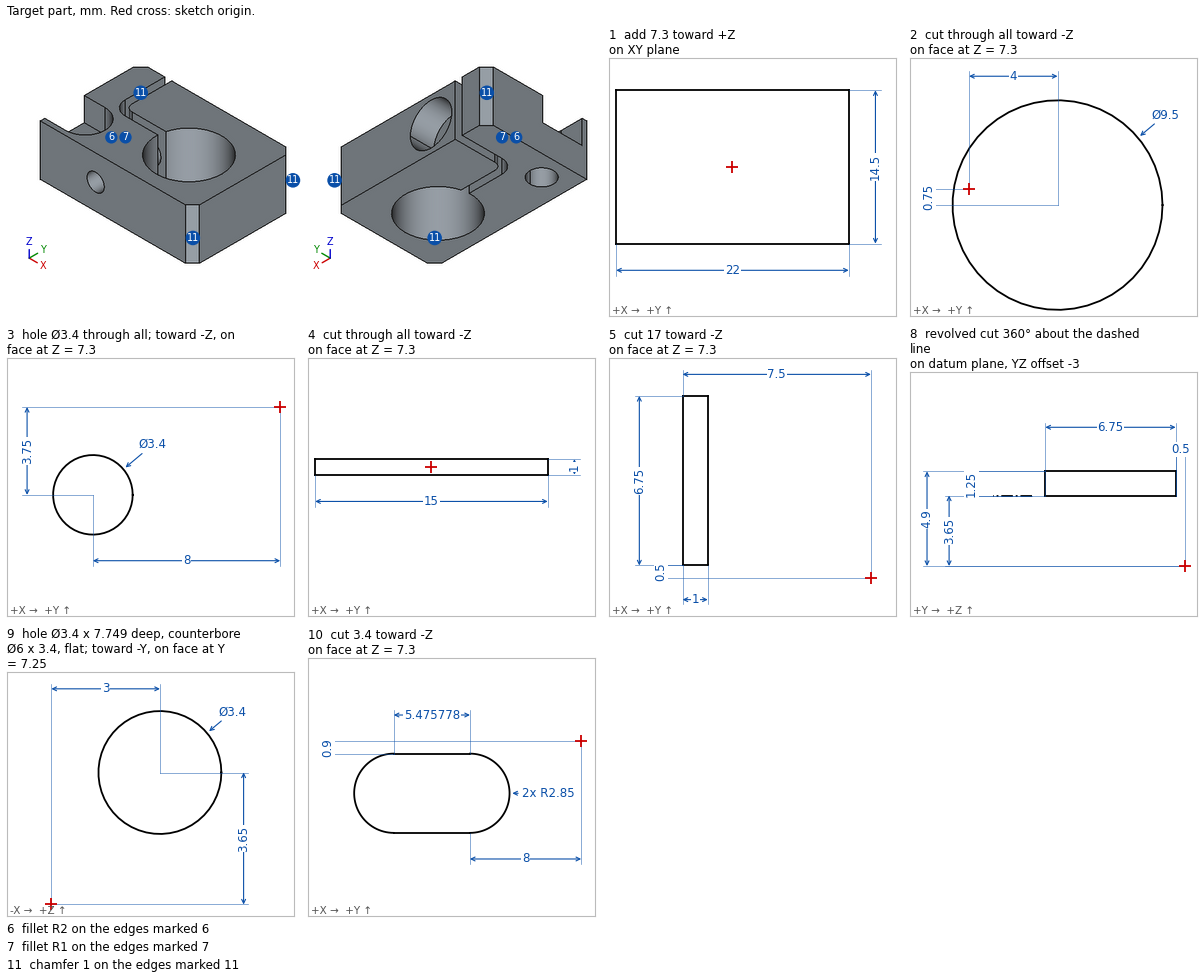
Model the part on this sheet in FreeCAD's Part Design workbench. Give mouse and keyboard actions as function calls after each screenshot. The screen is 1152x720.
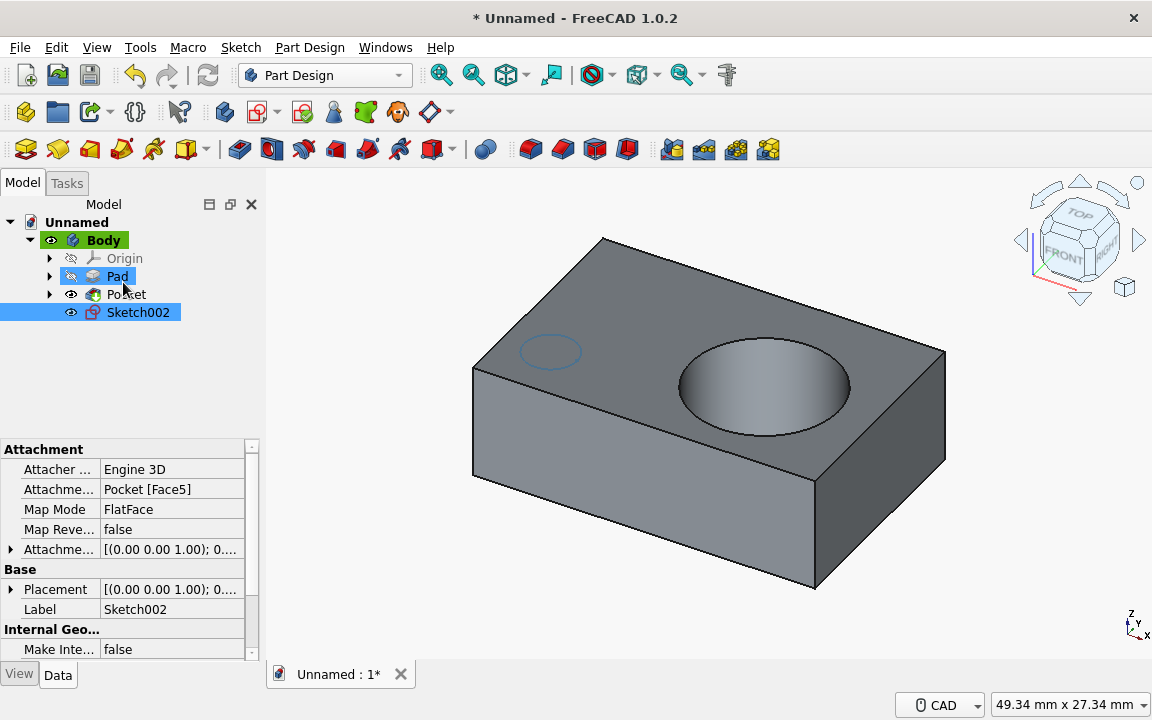
click(272, 150)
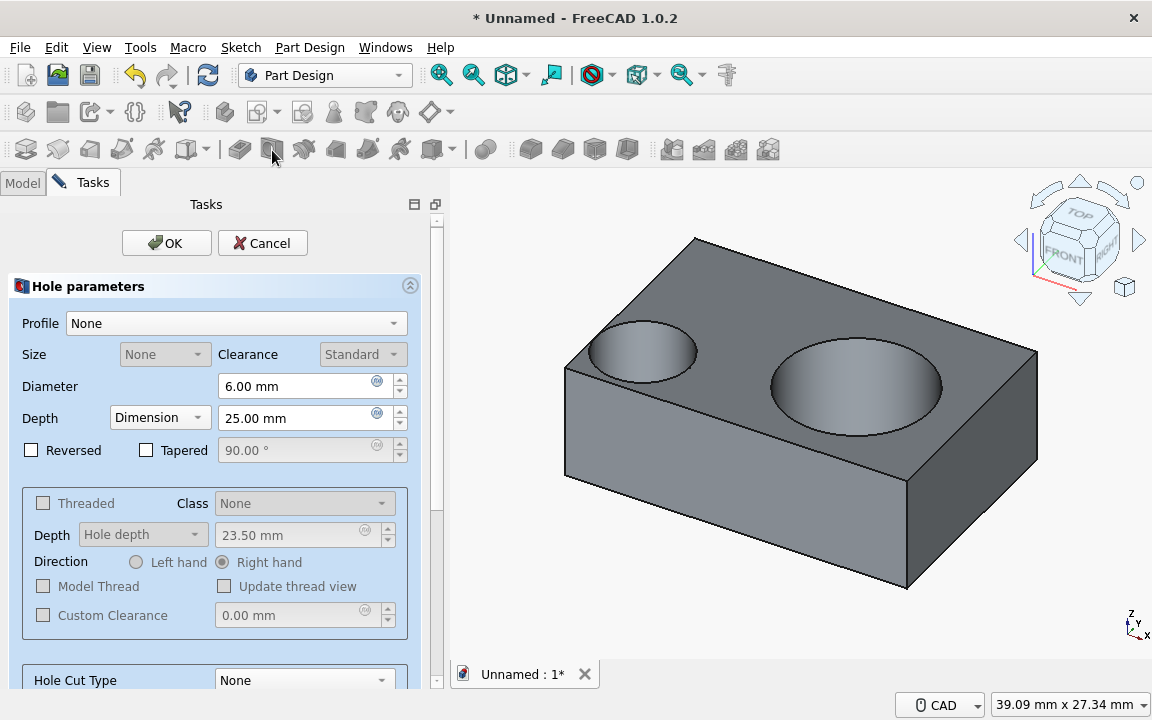
triple_click(305, 386)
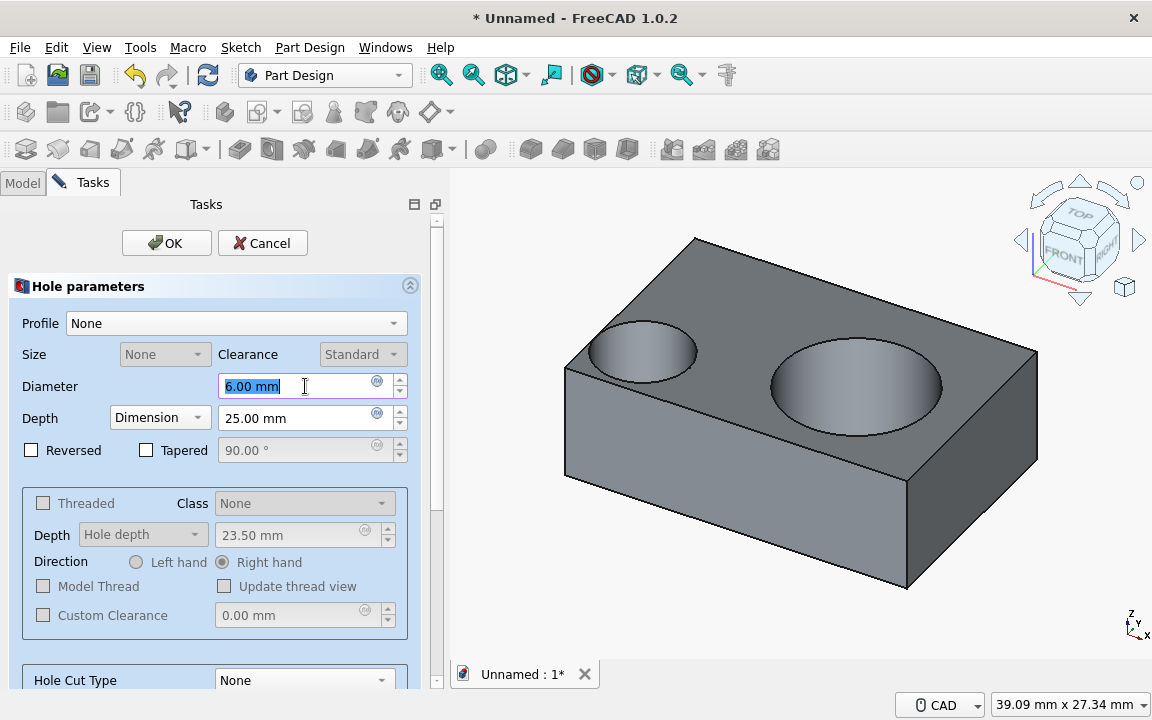
text(3.4)
key(Tab)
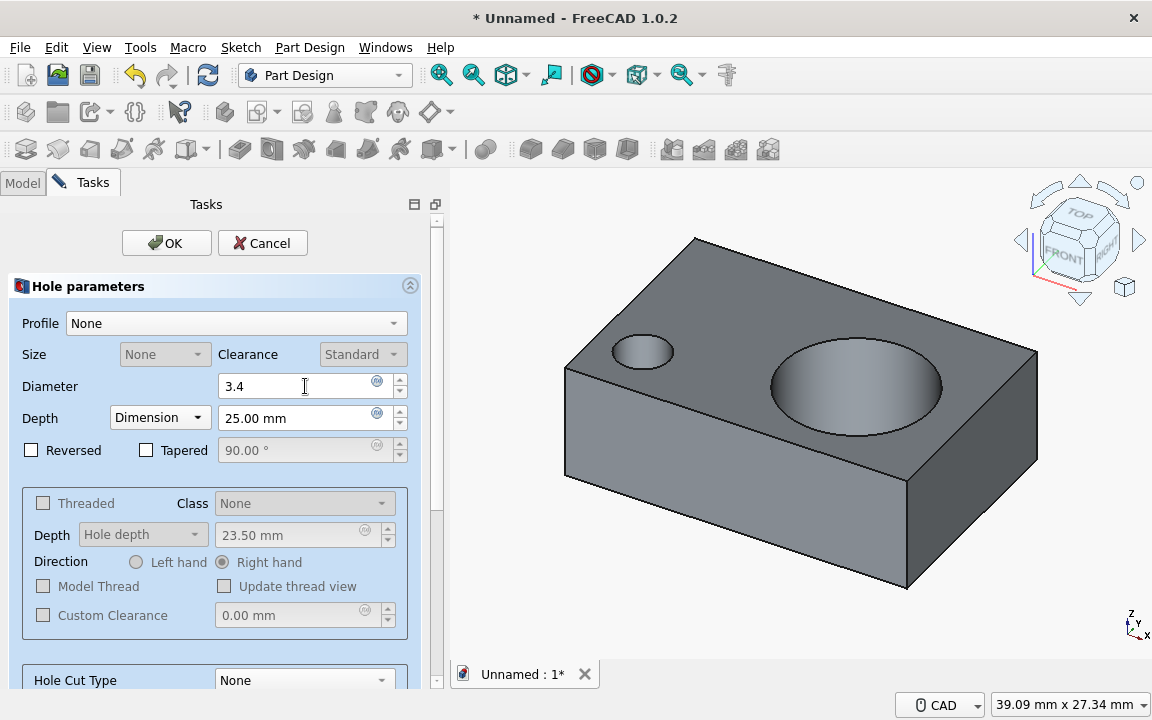
click(161, 418)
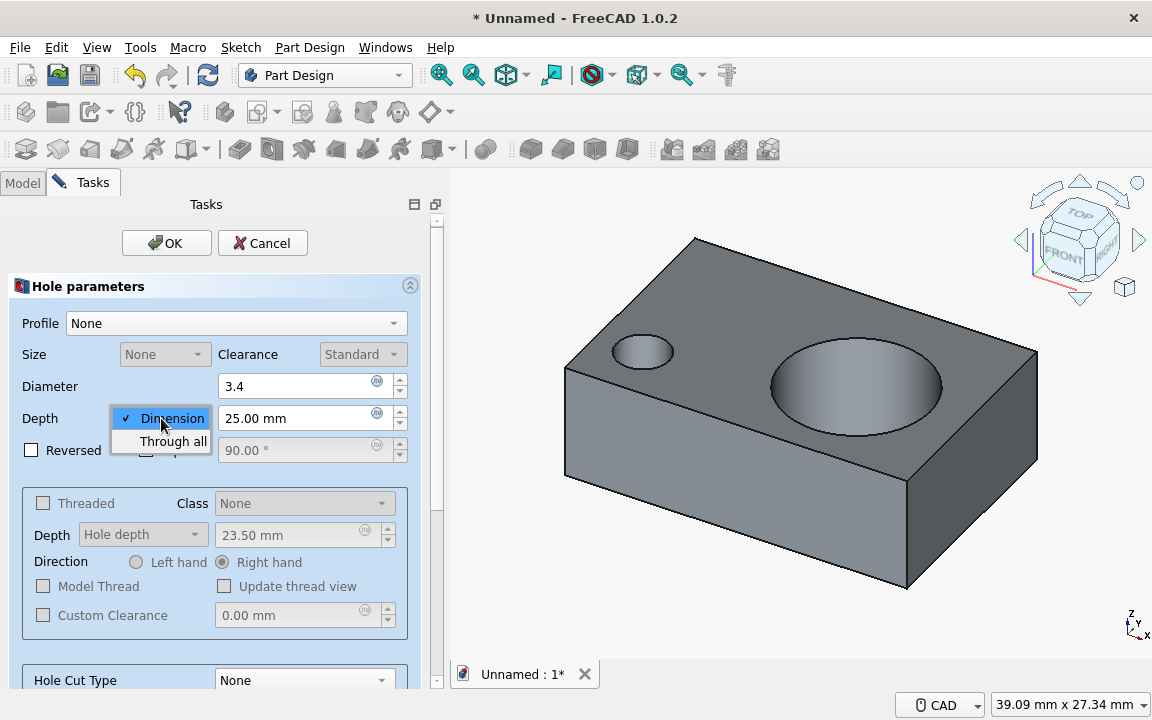
click(160, 442)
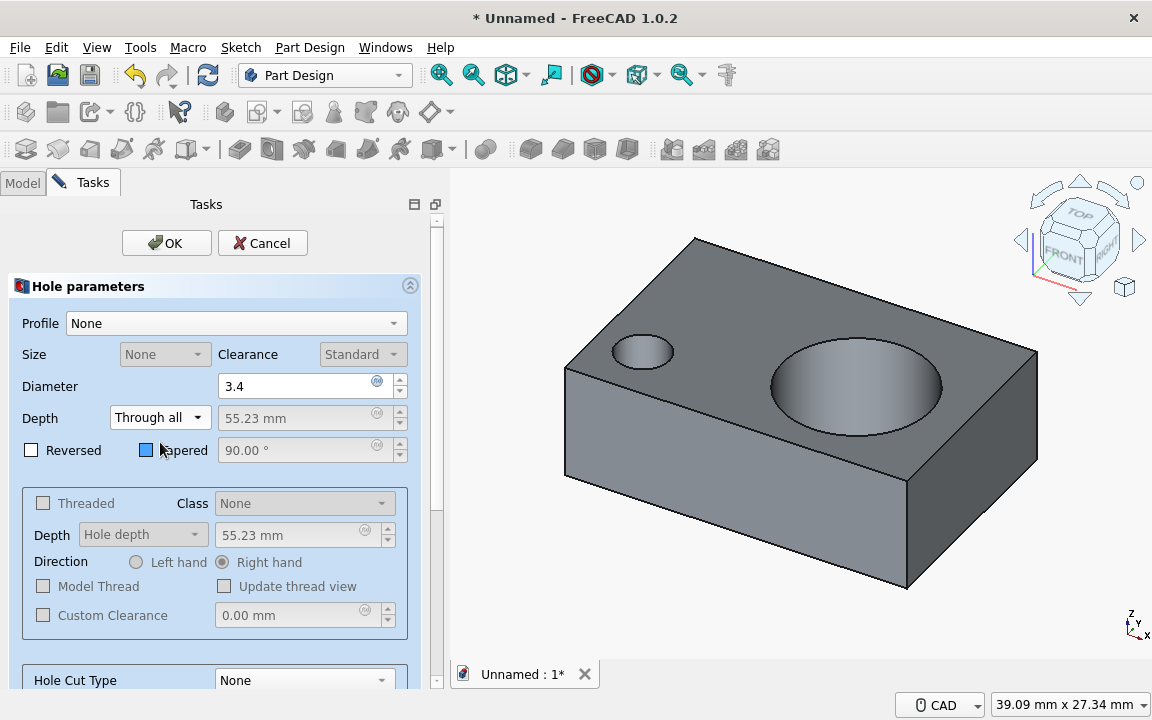
click(167, 243)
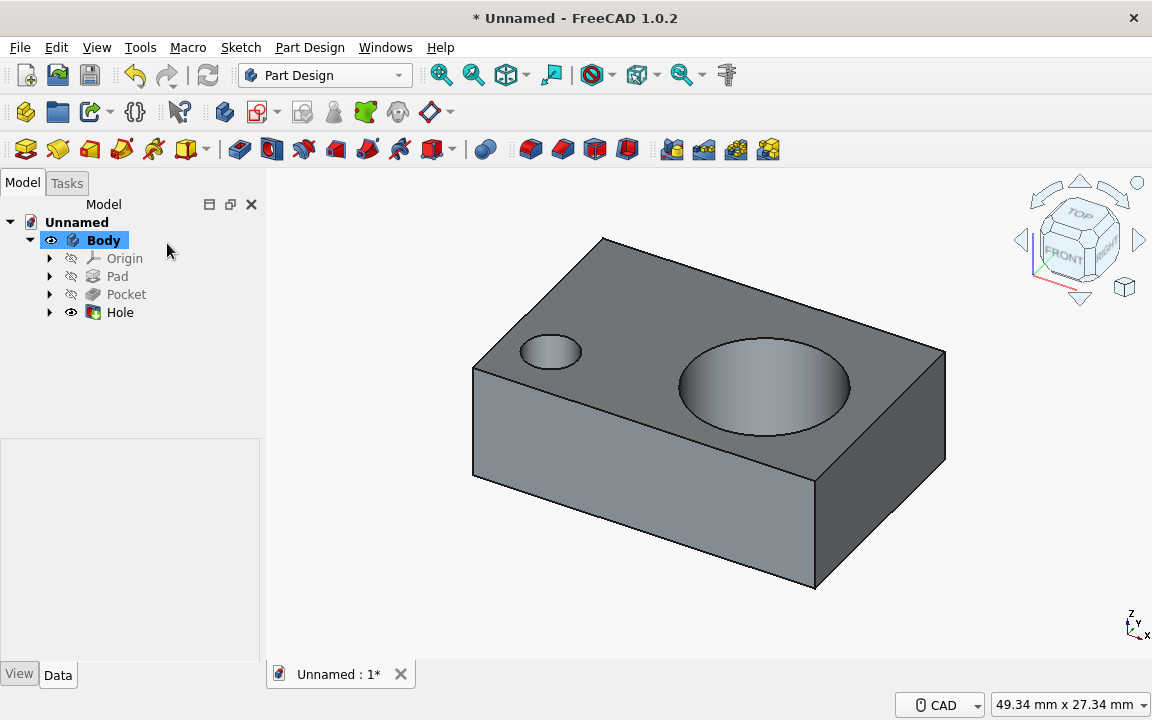
click(630, 308)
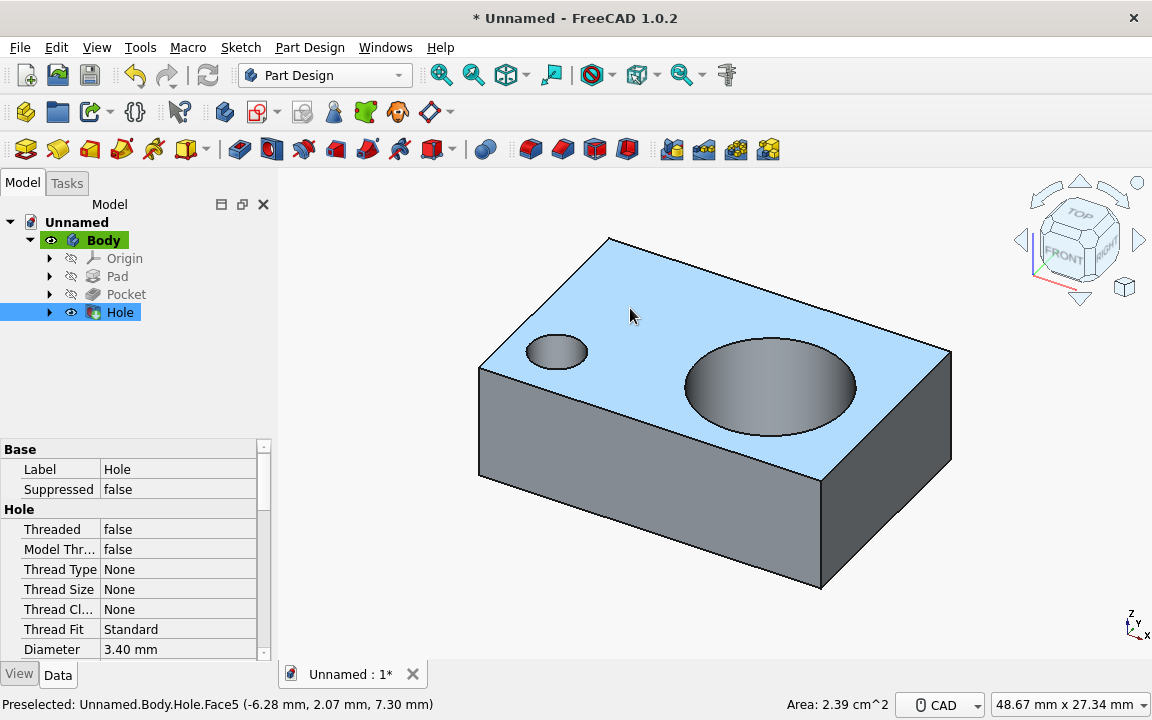
click(258, 112)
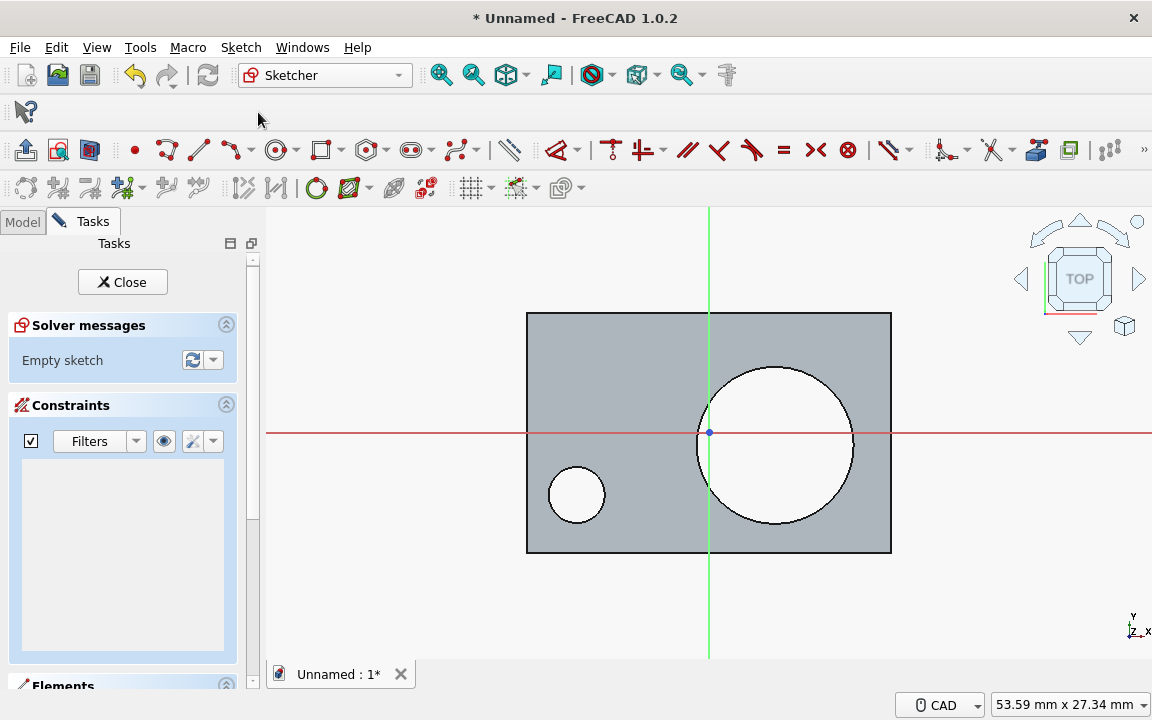
scroll(792, 433, up, 3)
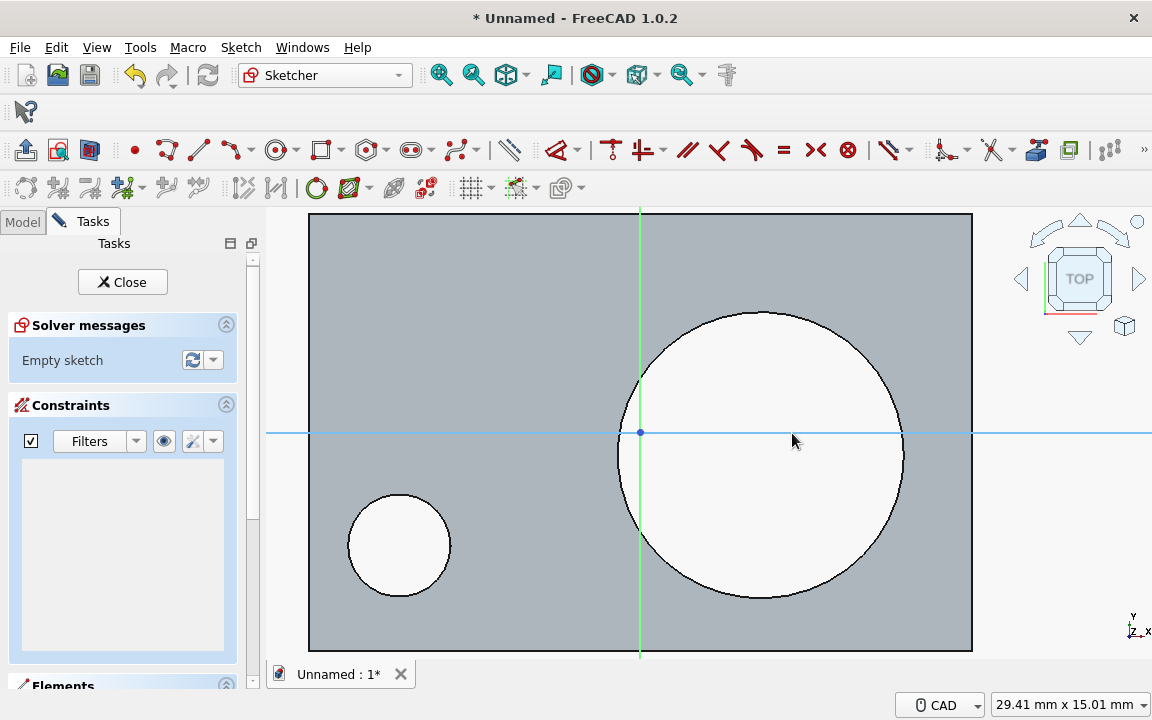
click(344, 150)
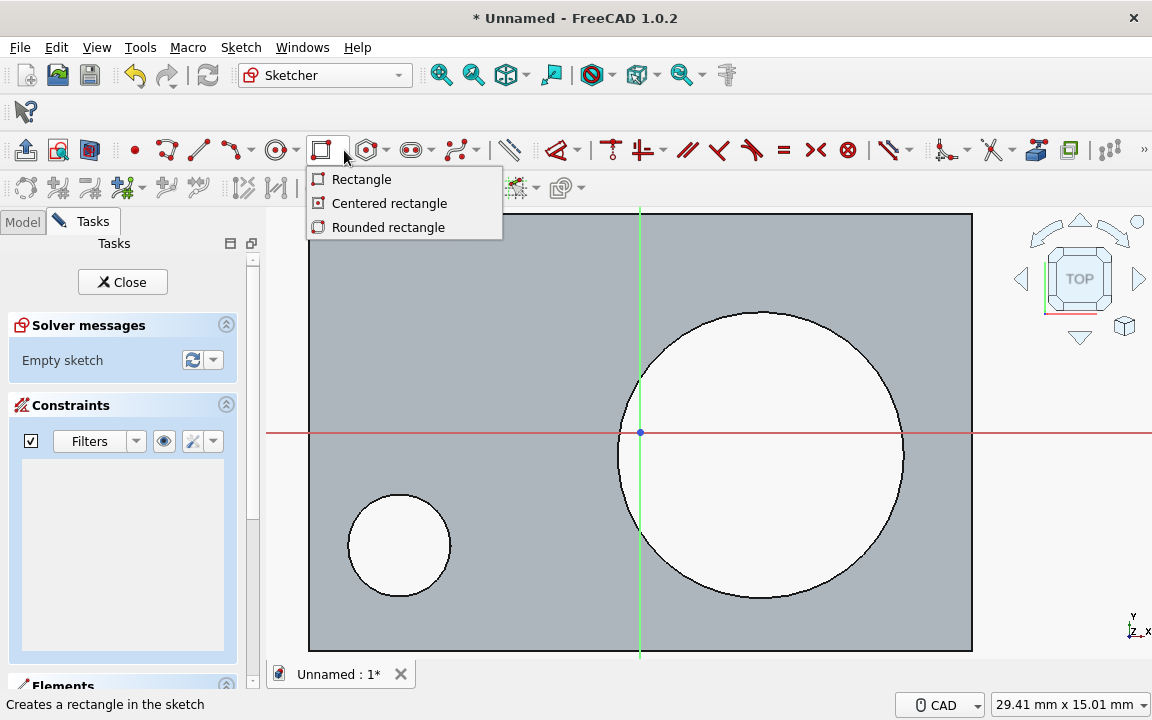
click(404, 203)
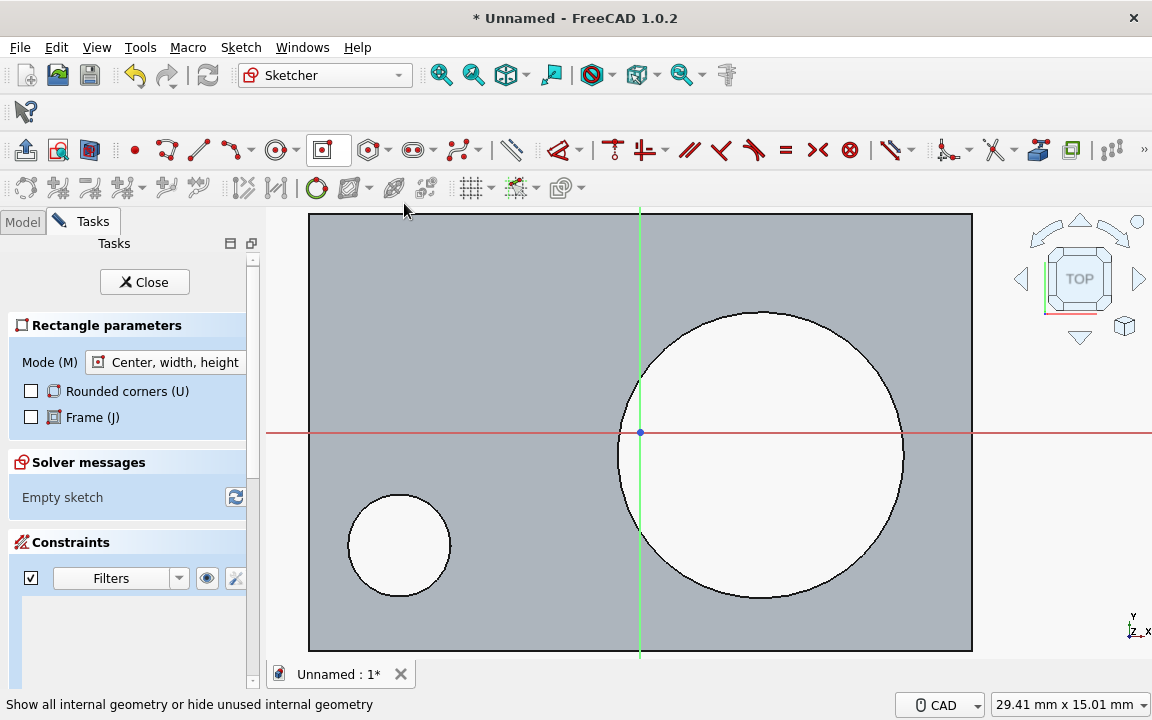
click(640, 433)
click(866, 418)
key(Escape)